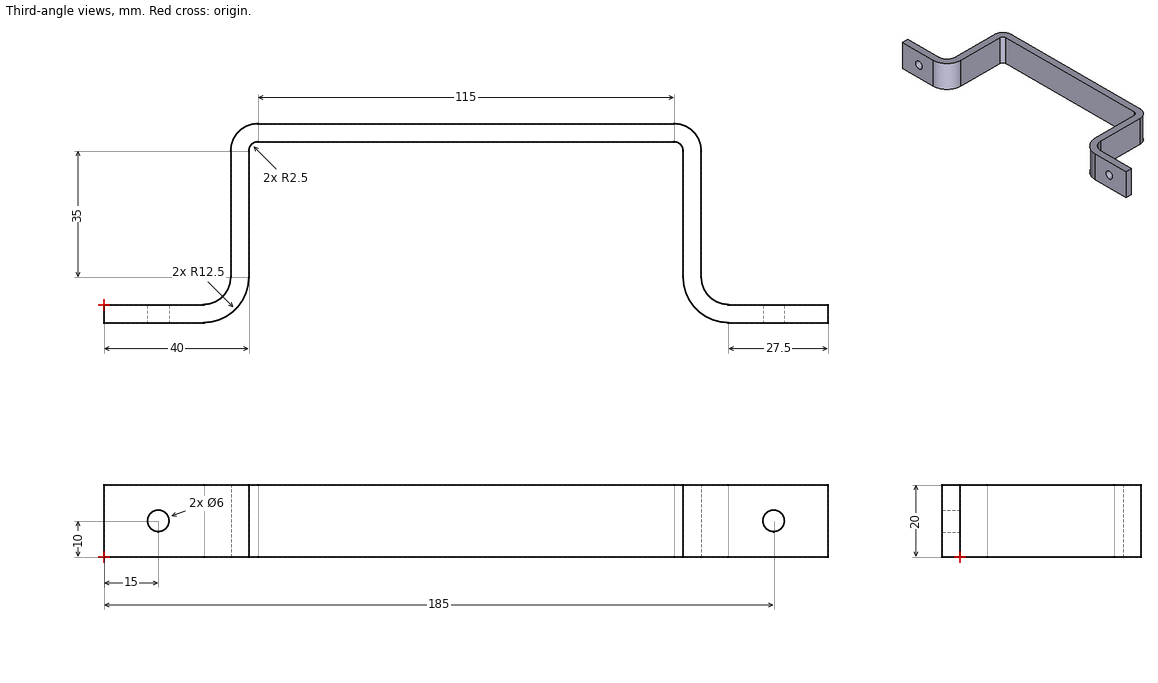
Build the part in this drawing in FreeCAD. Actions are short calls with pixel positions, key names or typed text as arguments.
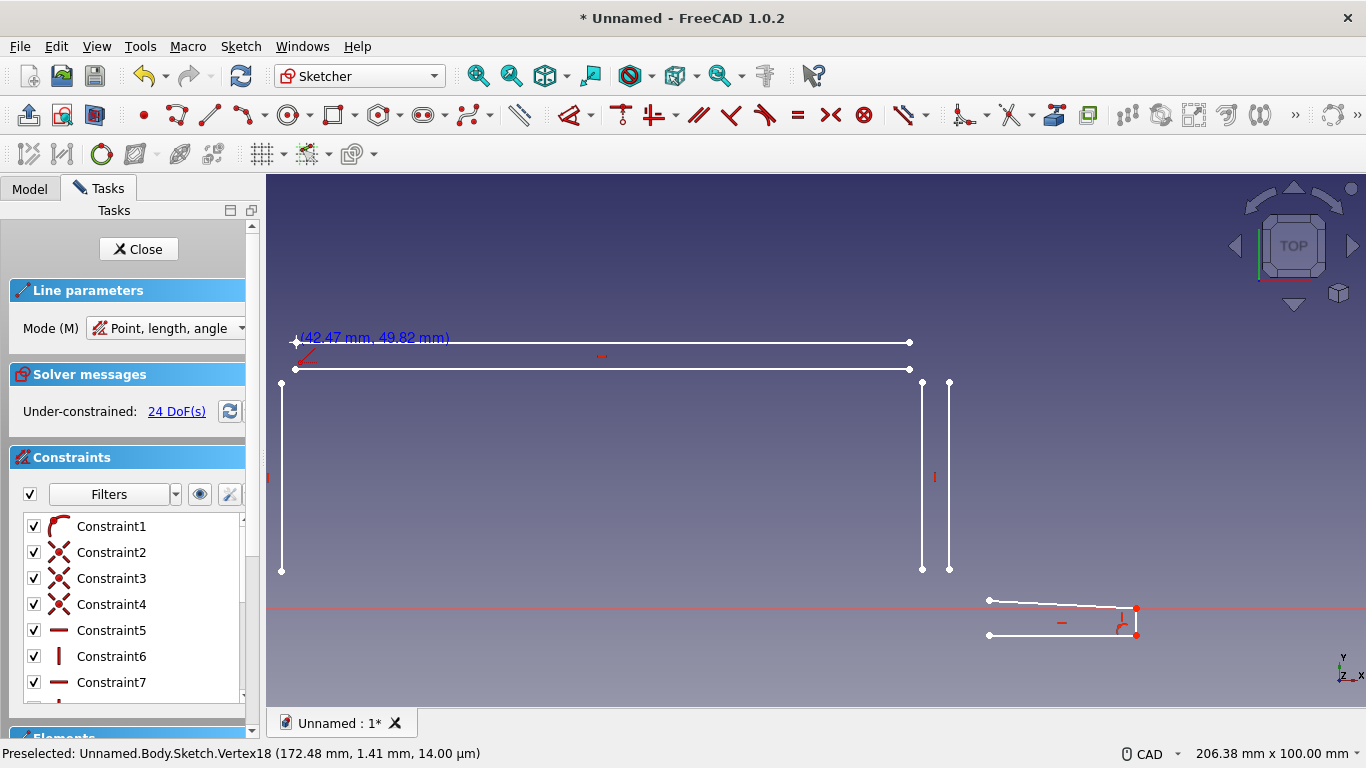
scroll(924, 382, down, 3)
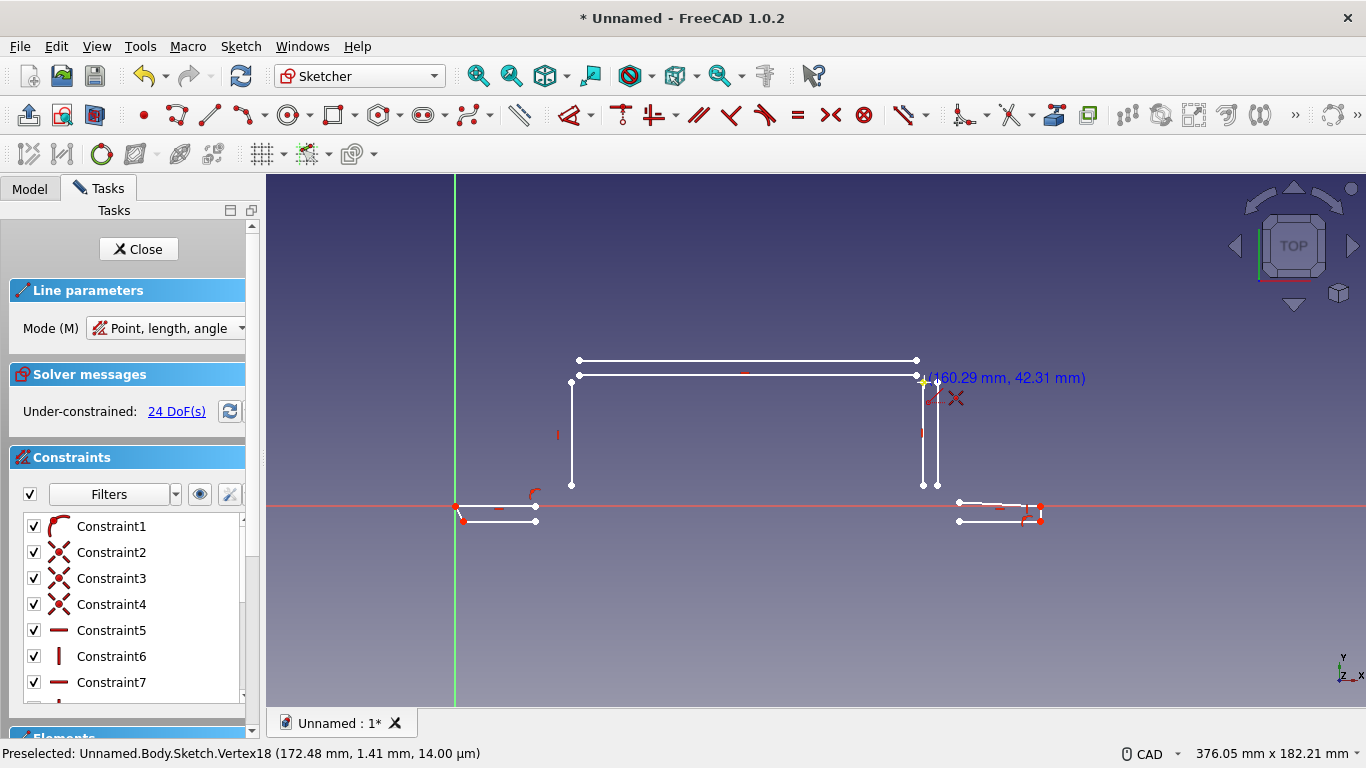
click(558, 382)
click(558, 485)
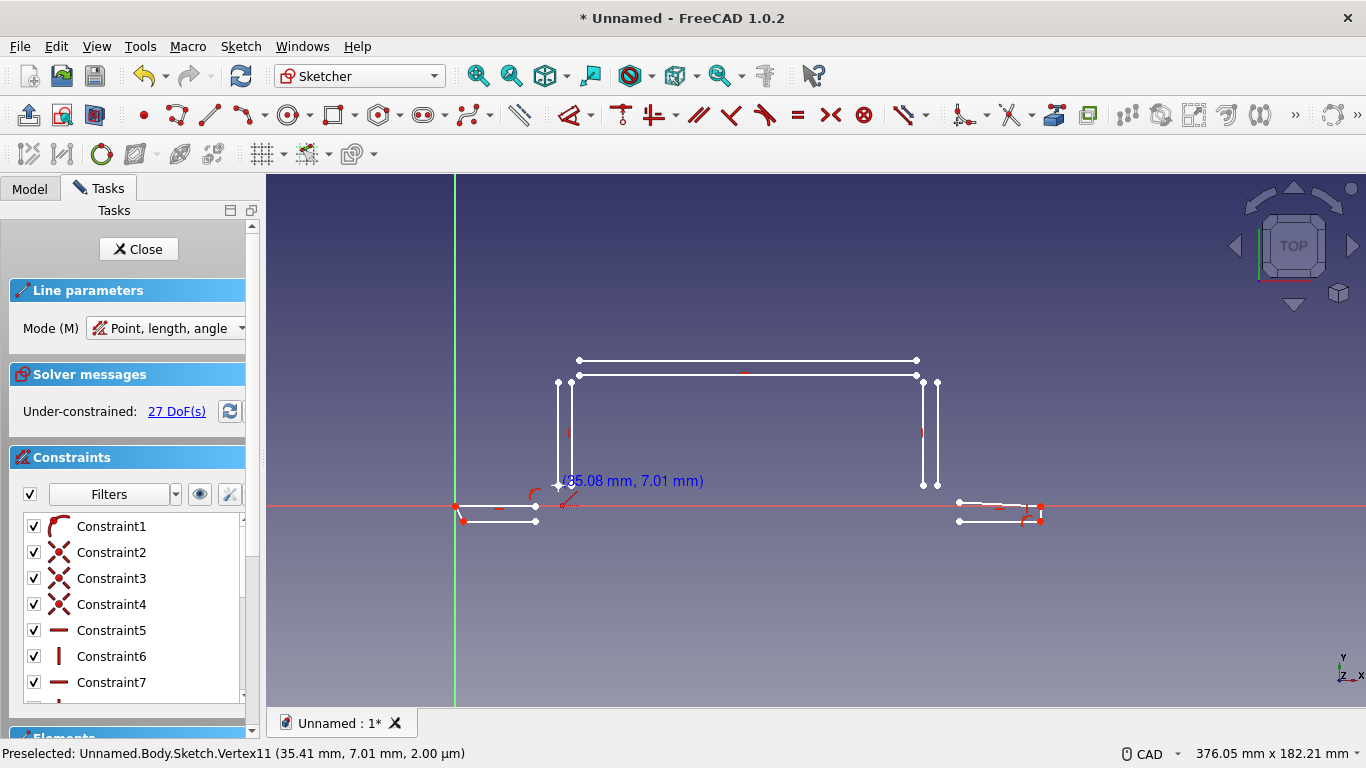
key(g)
key(3)
key(a)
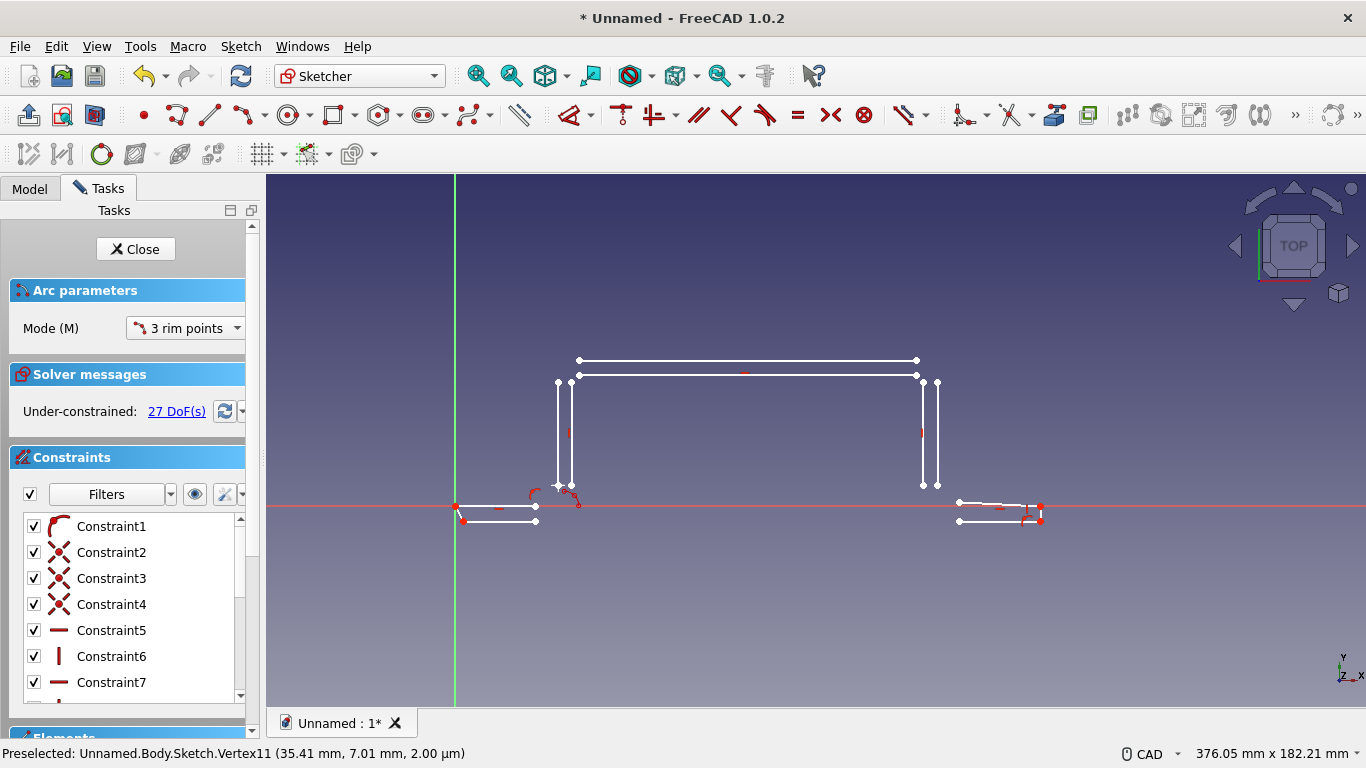
click(536, 522)
click(572, 486)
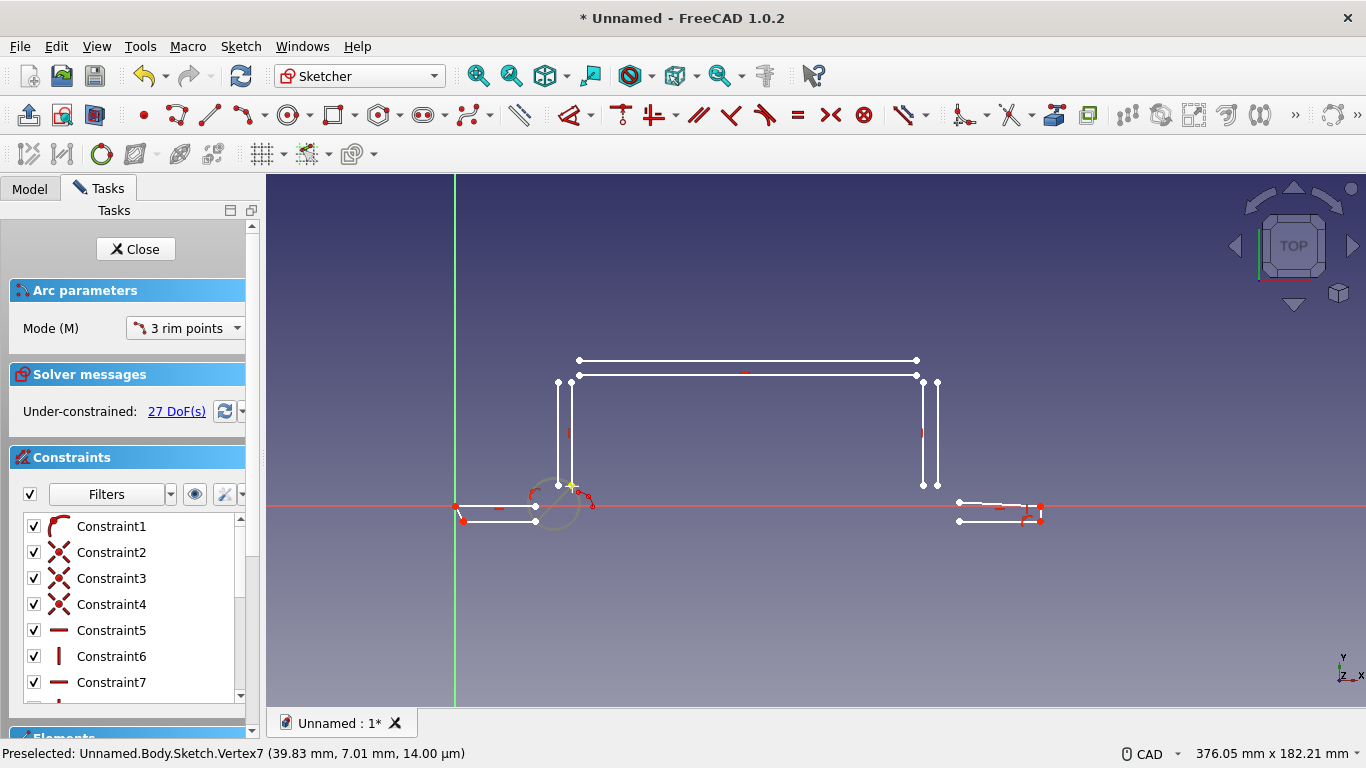
scroll(552, 517, up, 3)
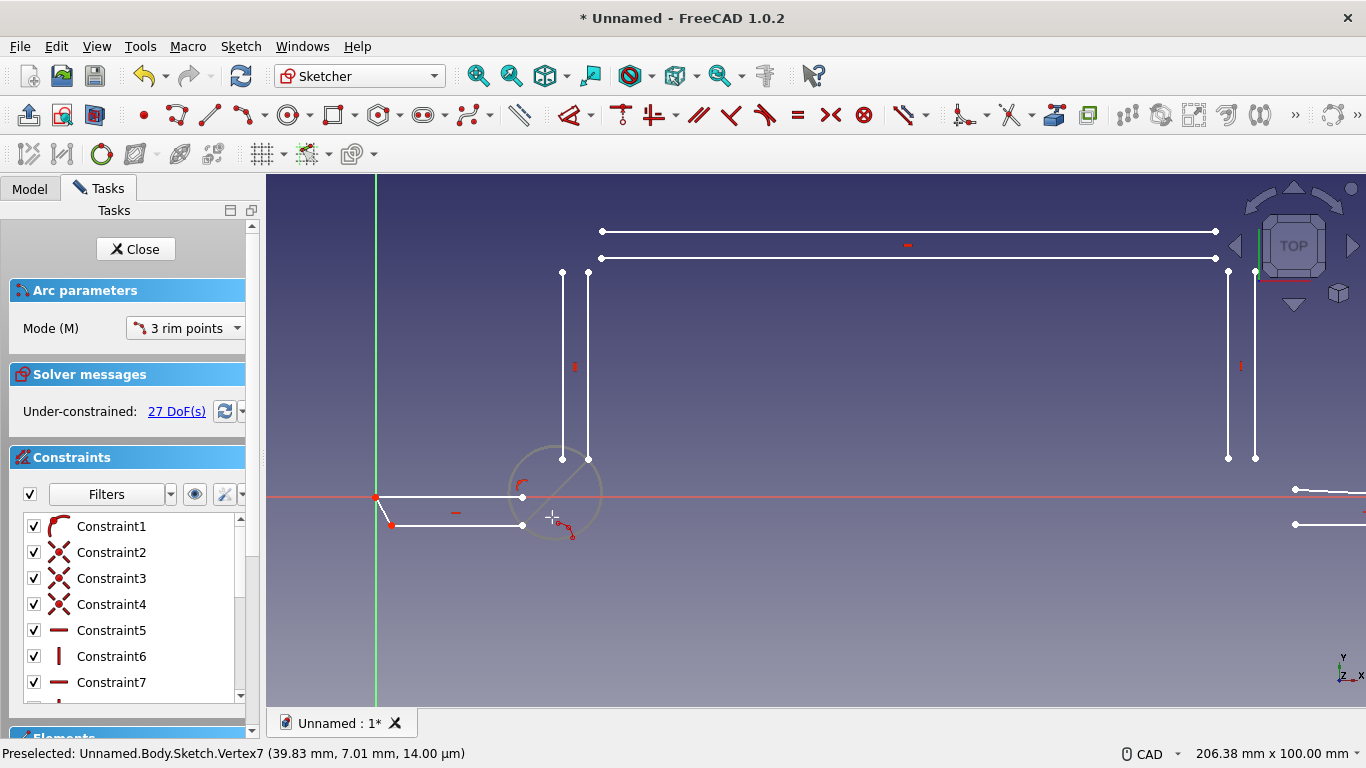
click(553, 517)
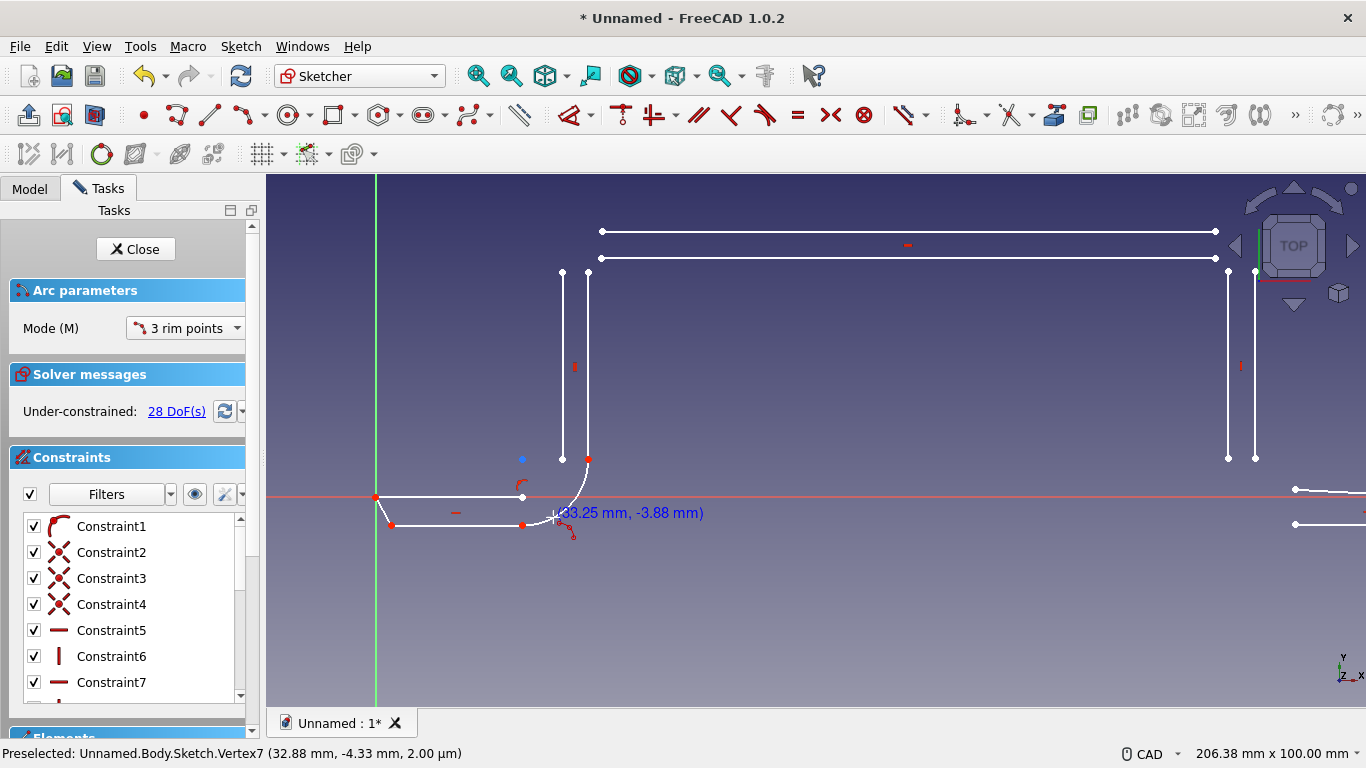
click(588, 272)
click(602, 258)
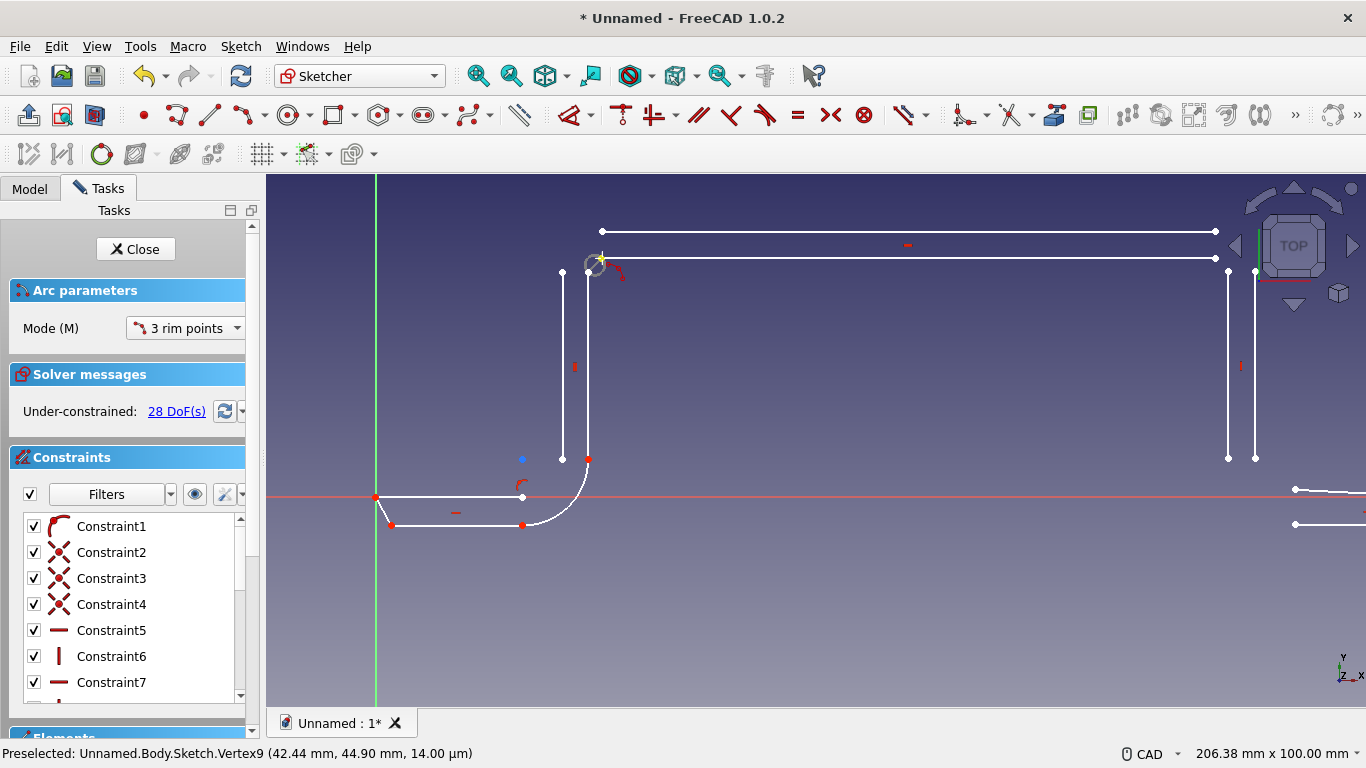
scroll(593, 261, up, 8)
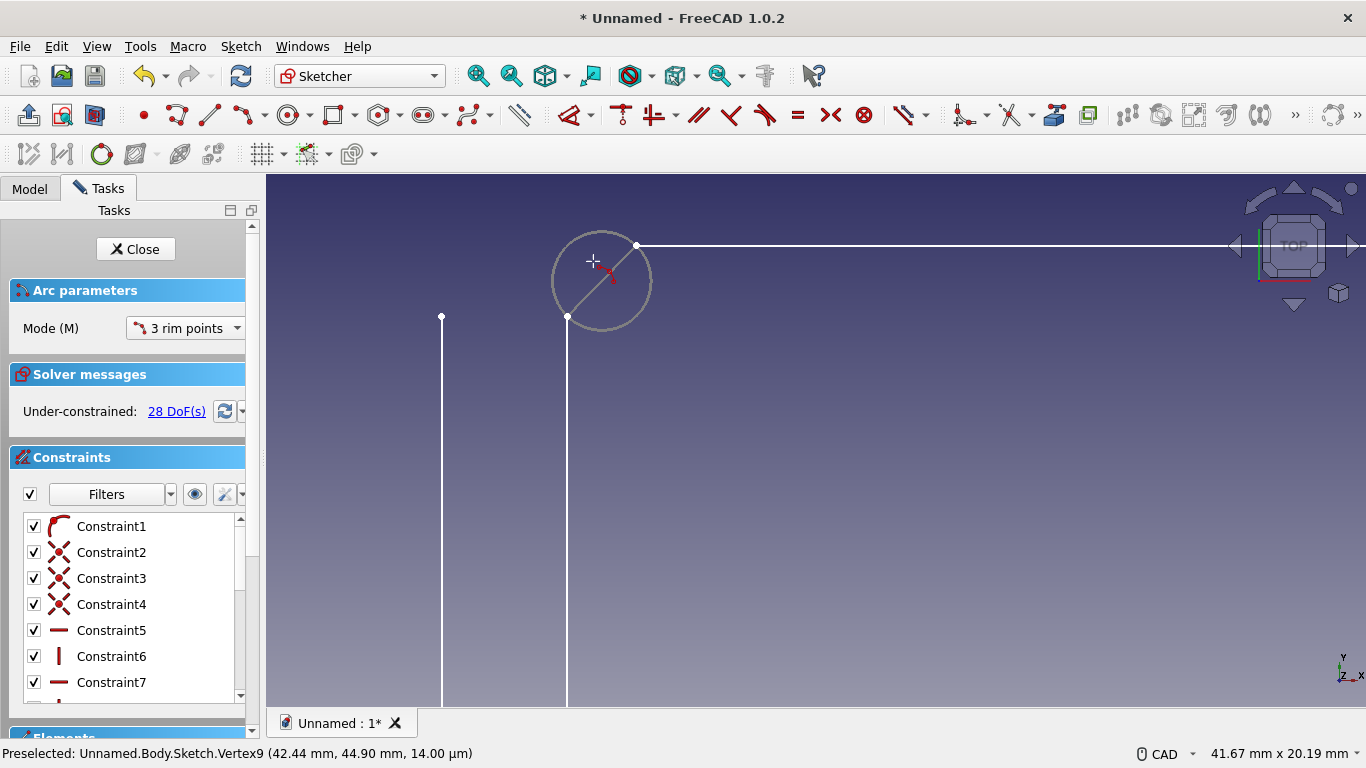
click(591, 262)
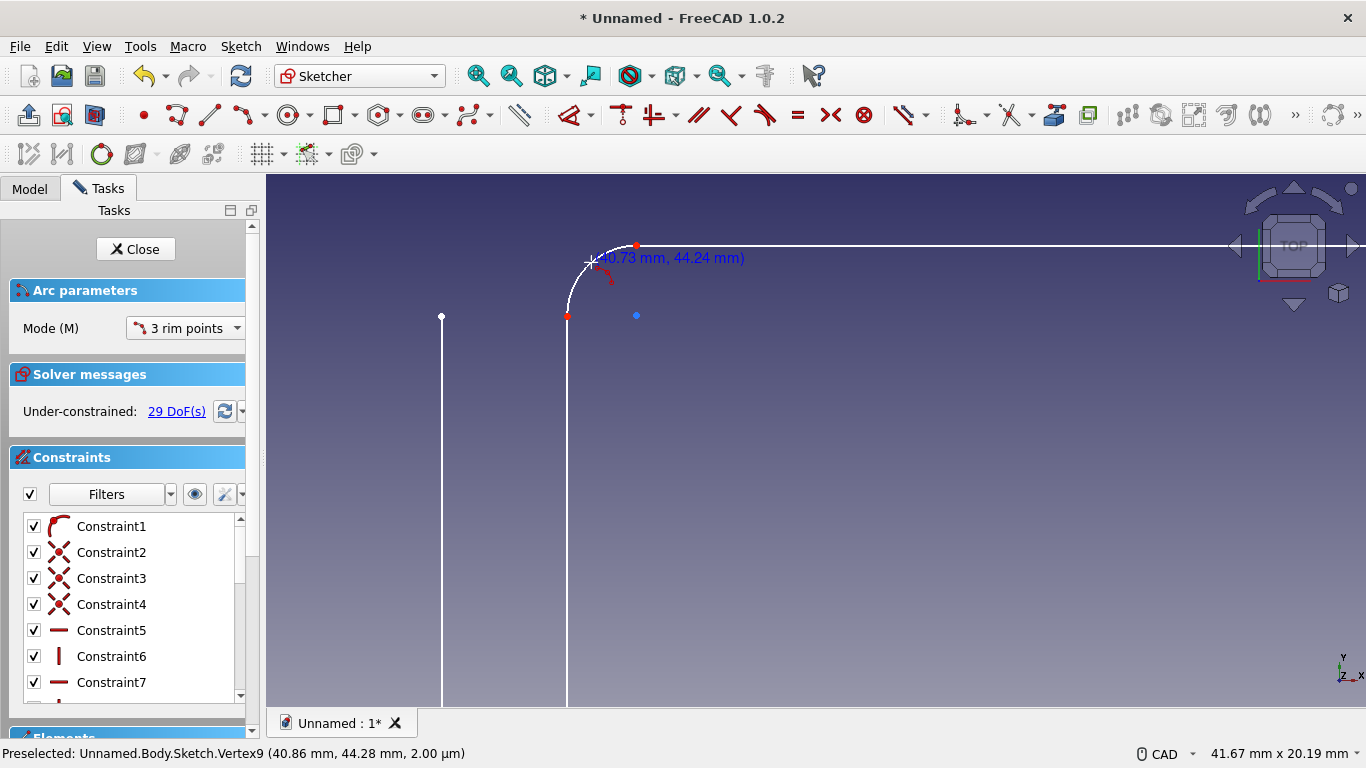
scroll(572, 391, down, 11)